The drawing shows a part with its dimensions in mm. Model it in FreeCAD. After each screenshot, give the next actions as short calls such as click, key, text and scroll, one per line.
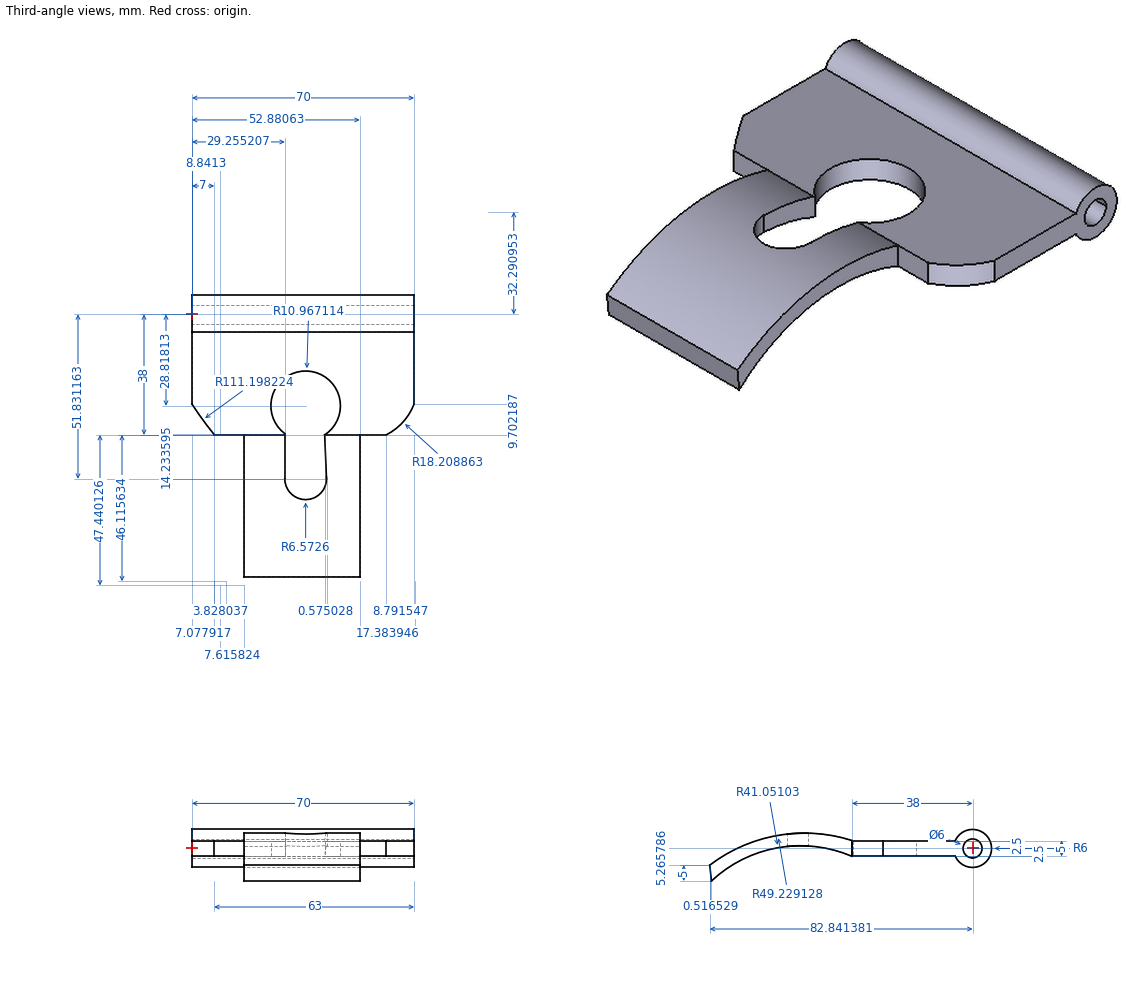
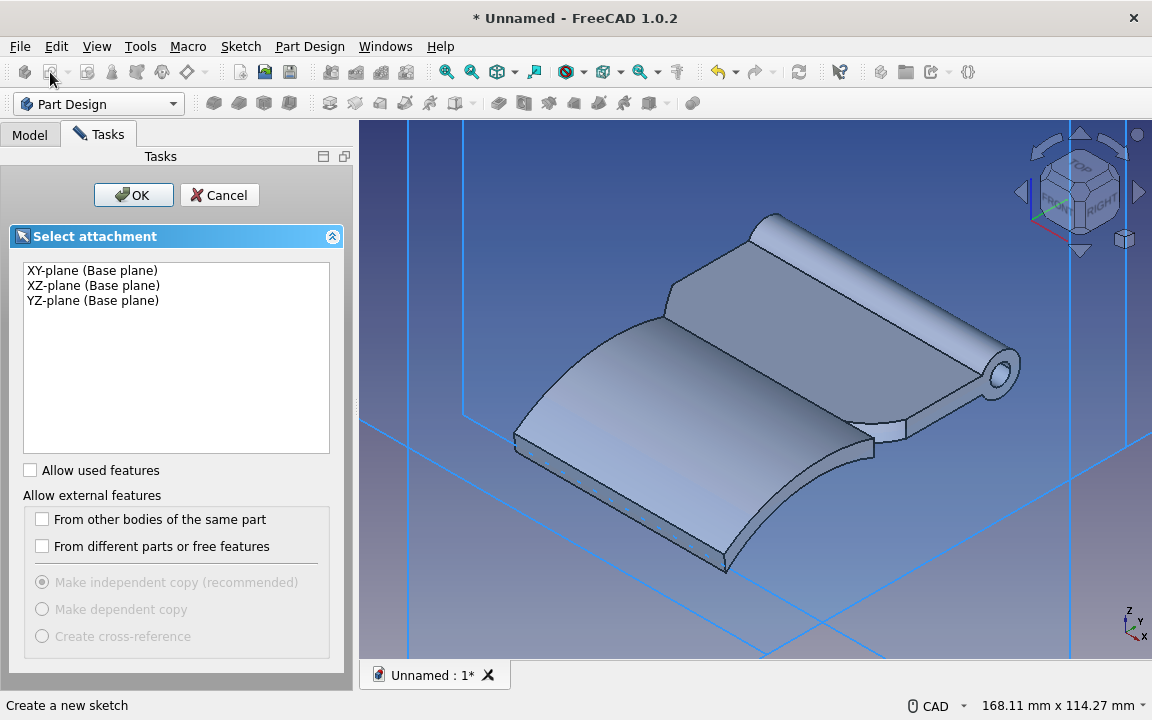
click(84, 270)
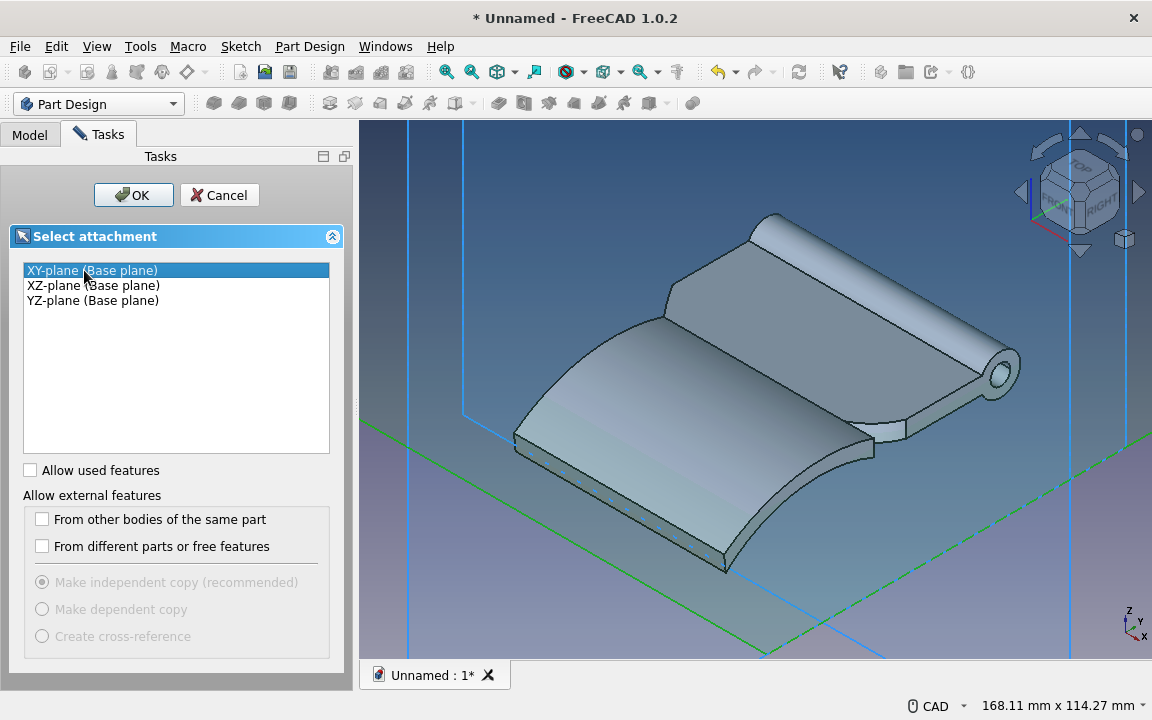
click(134, 195)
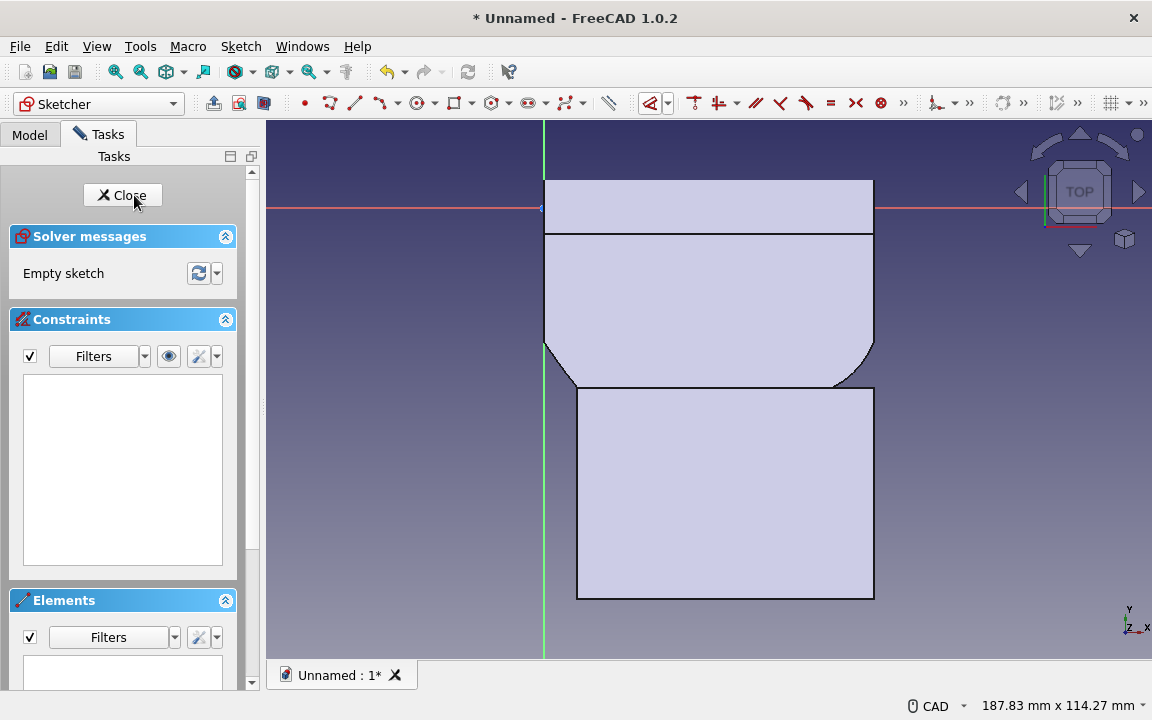
click(264, 104)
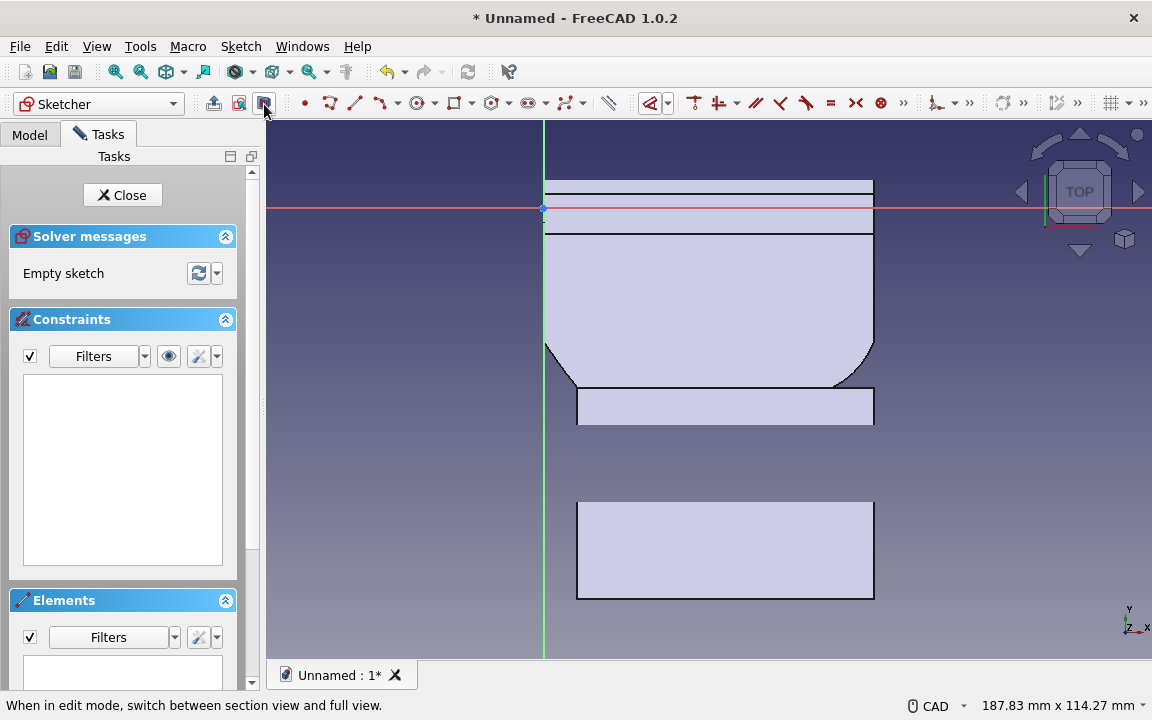
click(454, 104)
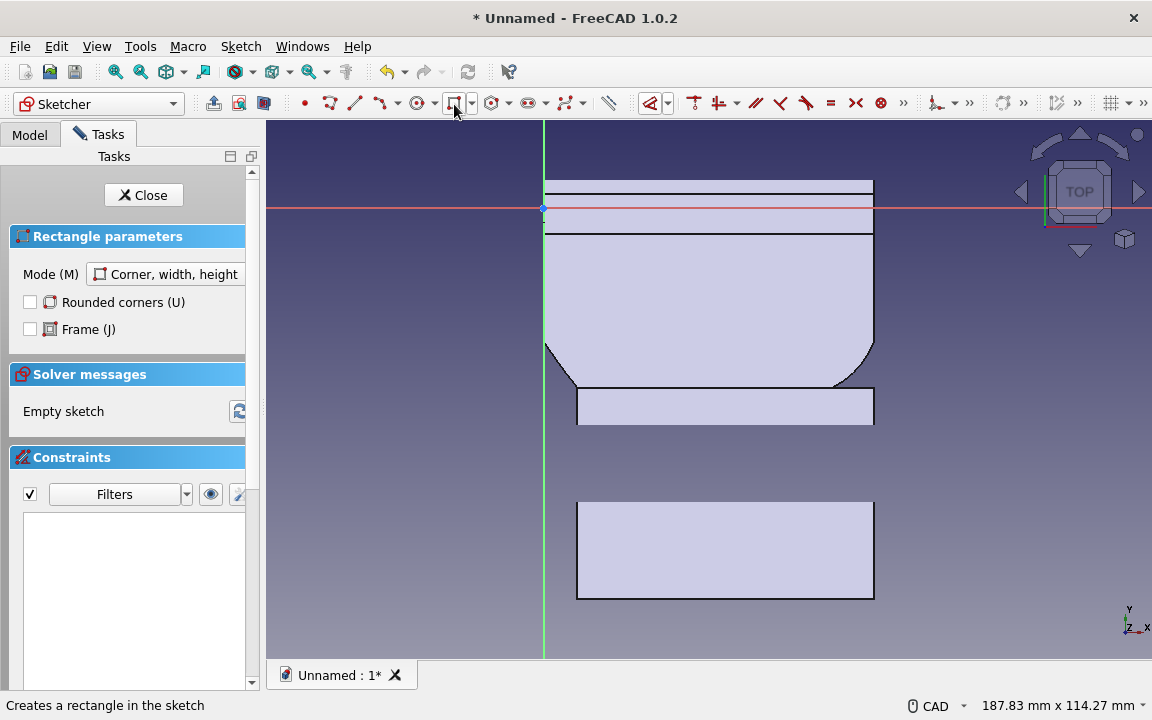
click(577, 388)
move(595, 605)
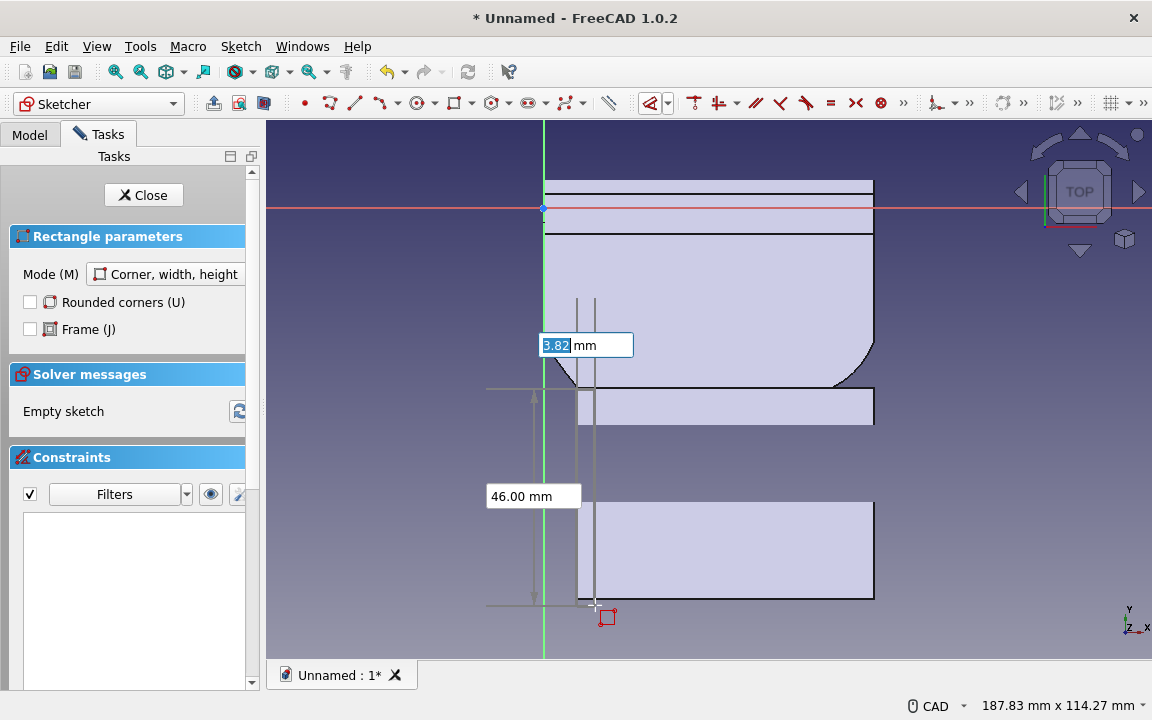
text(3.828037)
key(Tab)
text(46.115634)
key(Return)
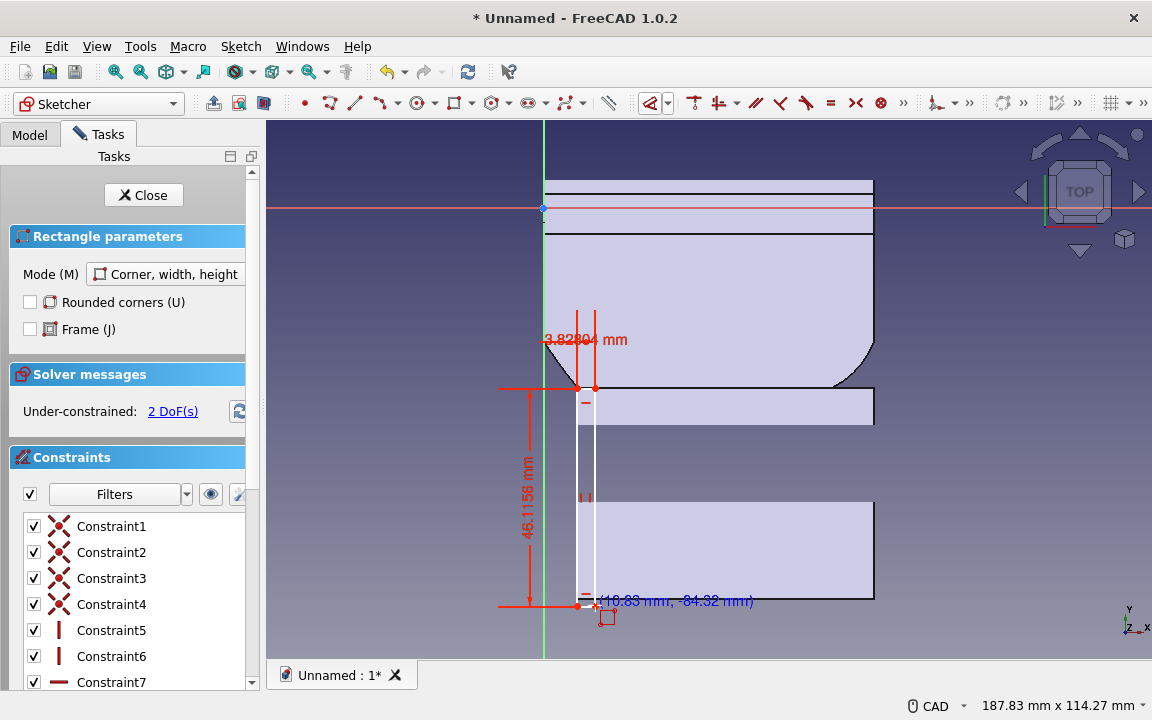
click(793, 388)
move(875, 605)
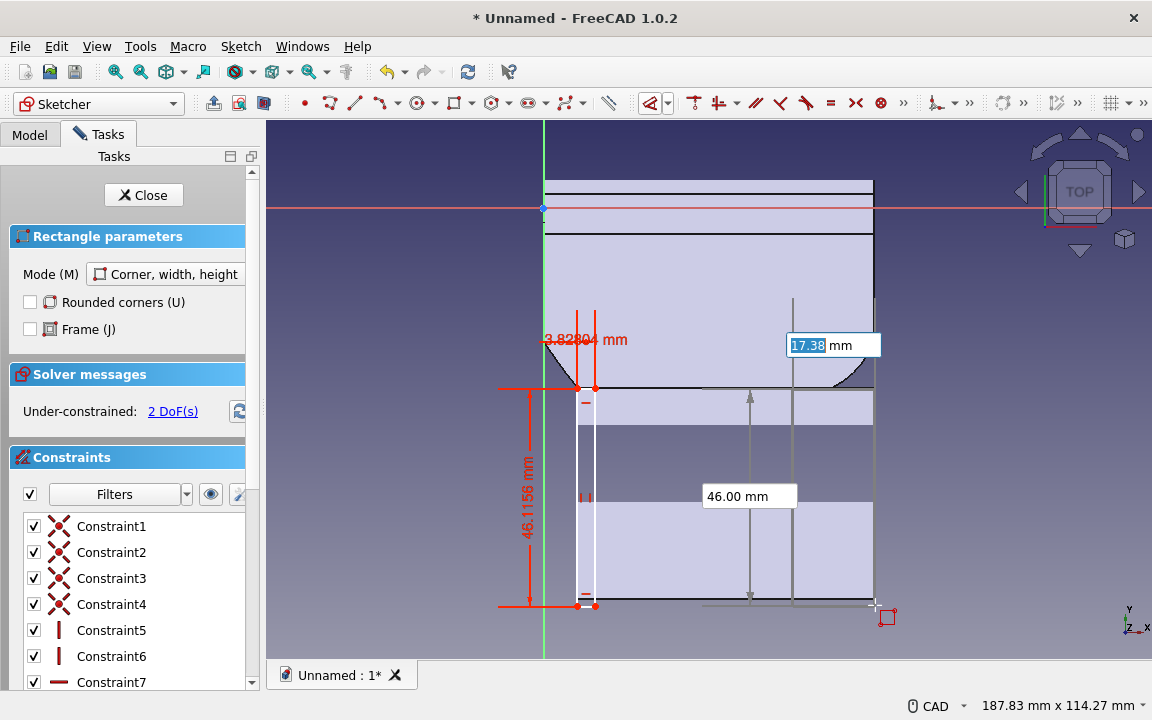
text(17.383946)
key(Tab)
text(46.115634)
key(Return)
key(Escape)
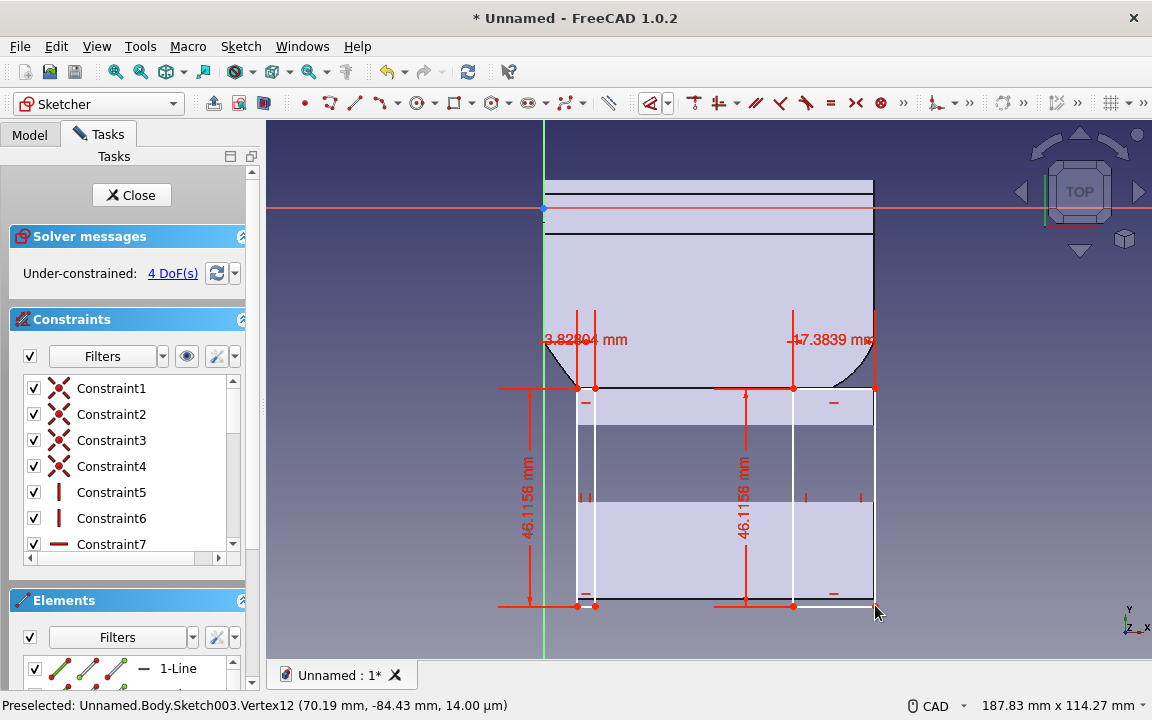
click(577, 389)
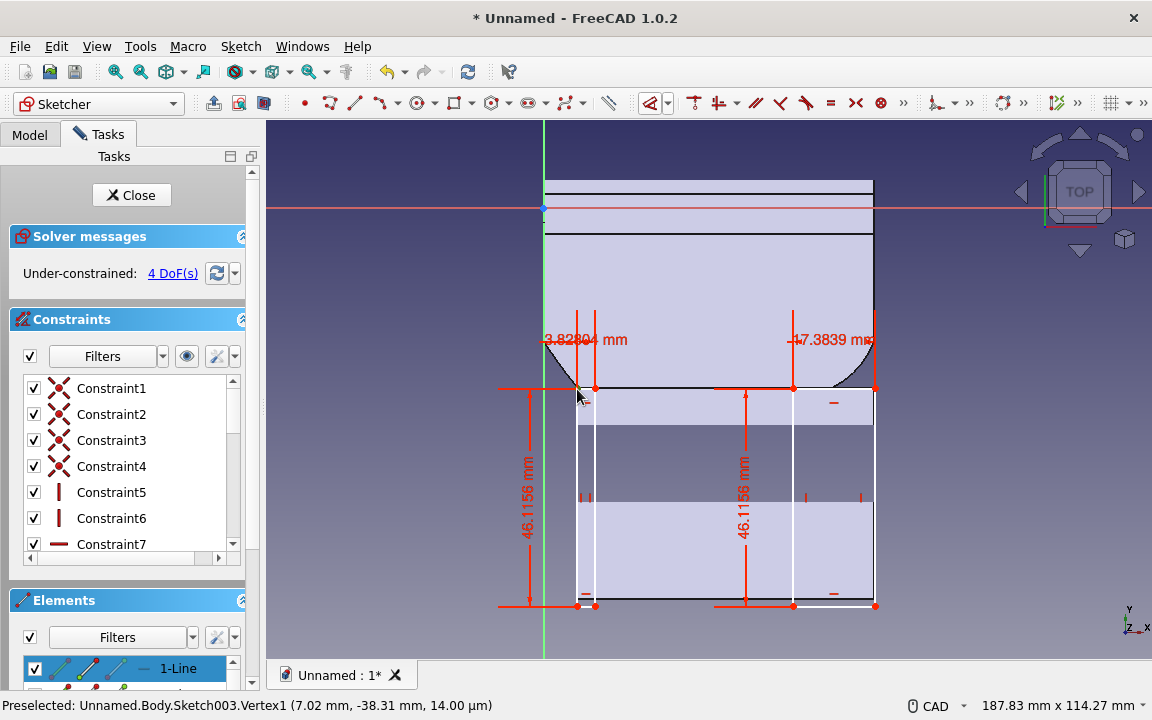
click(668, 104)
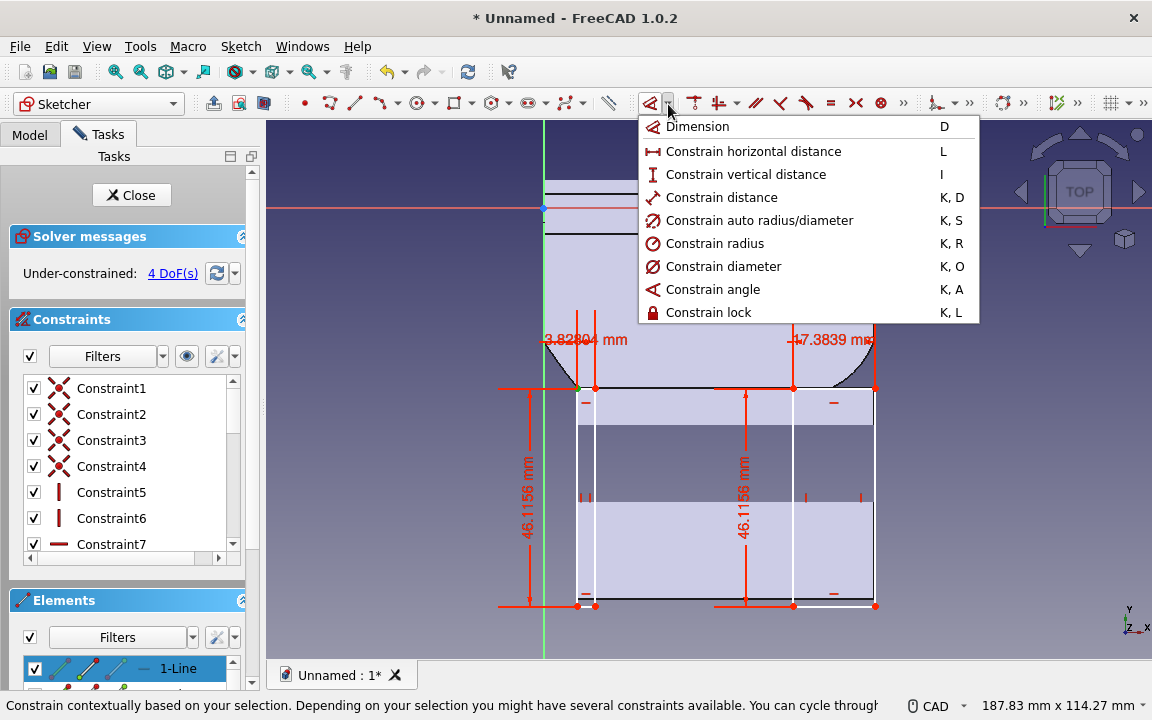
click(809, 152)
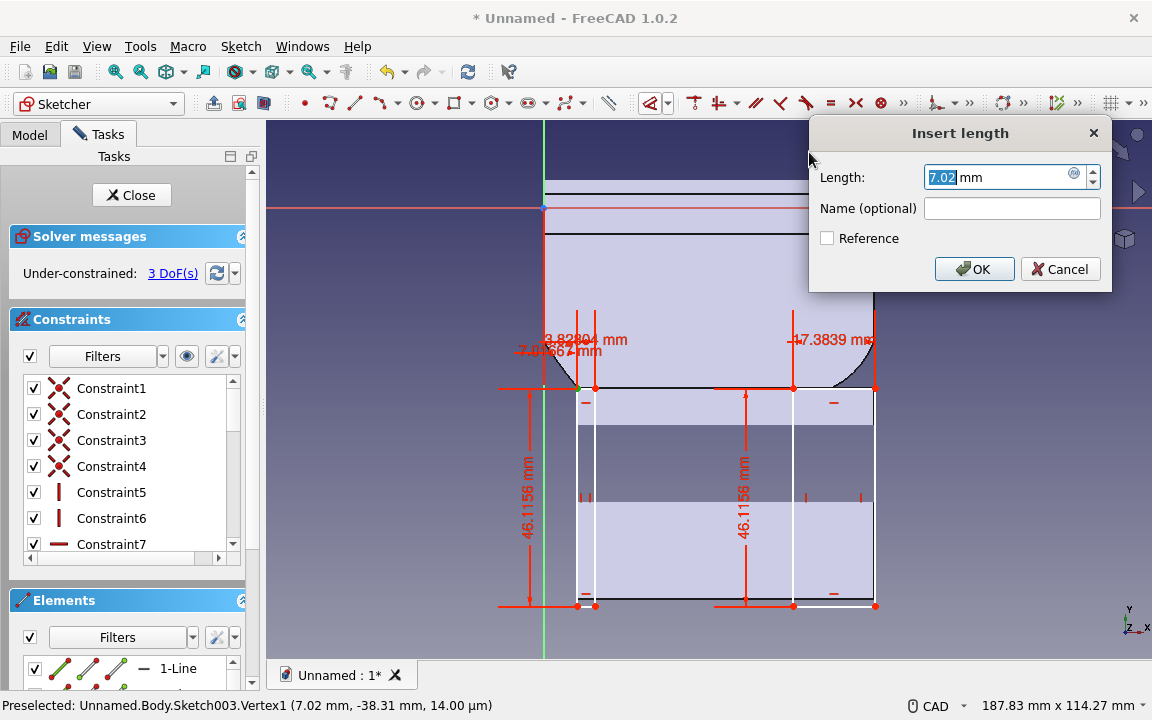
text(7)
key(Return)